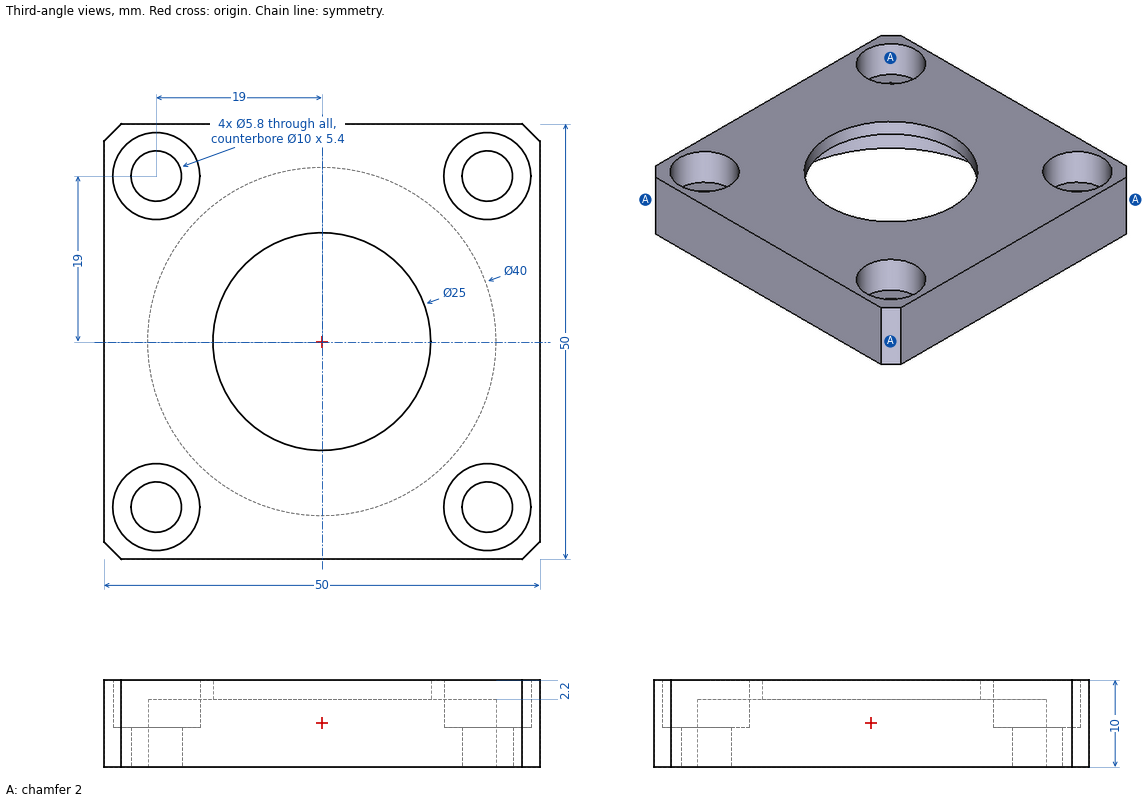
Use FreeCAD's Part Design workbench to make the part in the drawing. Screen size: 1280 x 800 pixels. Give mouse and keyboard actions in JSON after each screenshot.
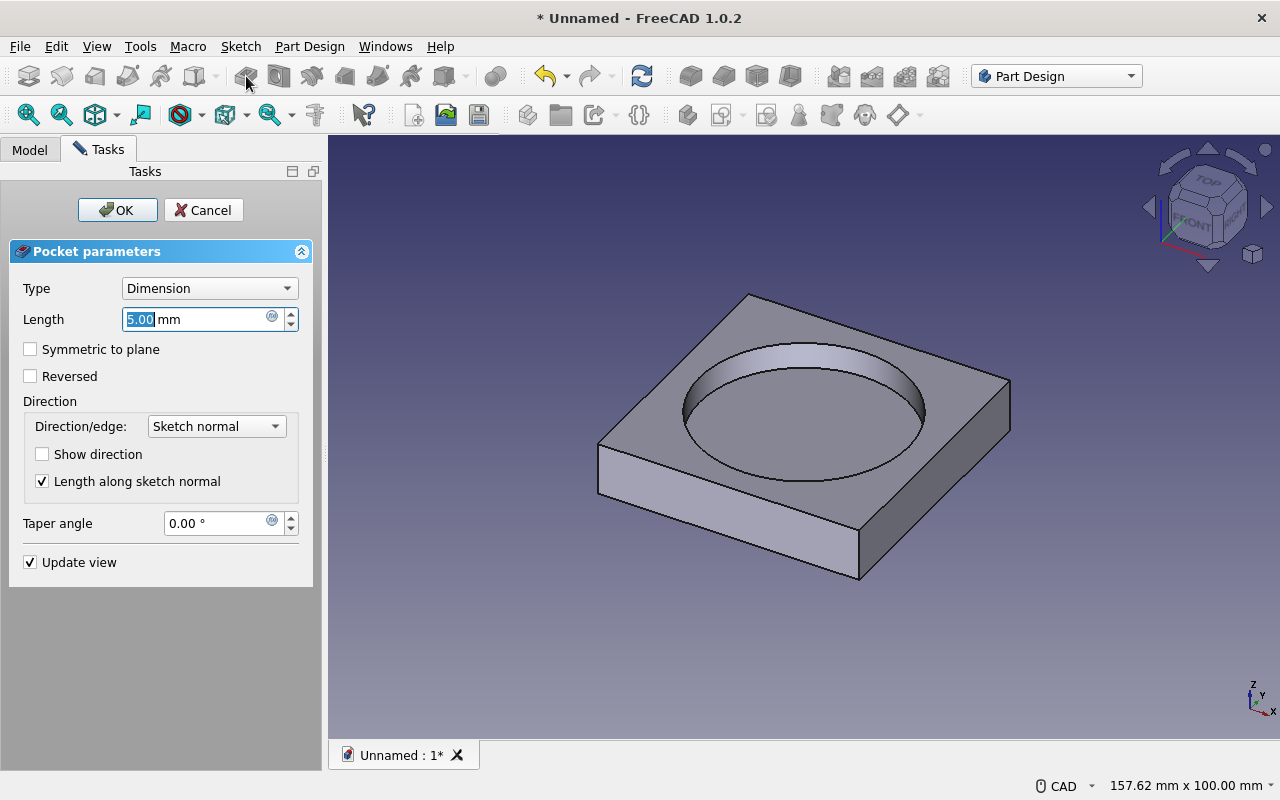
{"action": "left_click", "coordinate": [210, 288]}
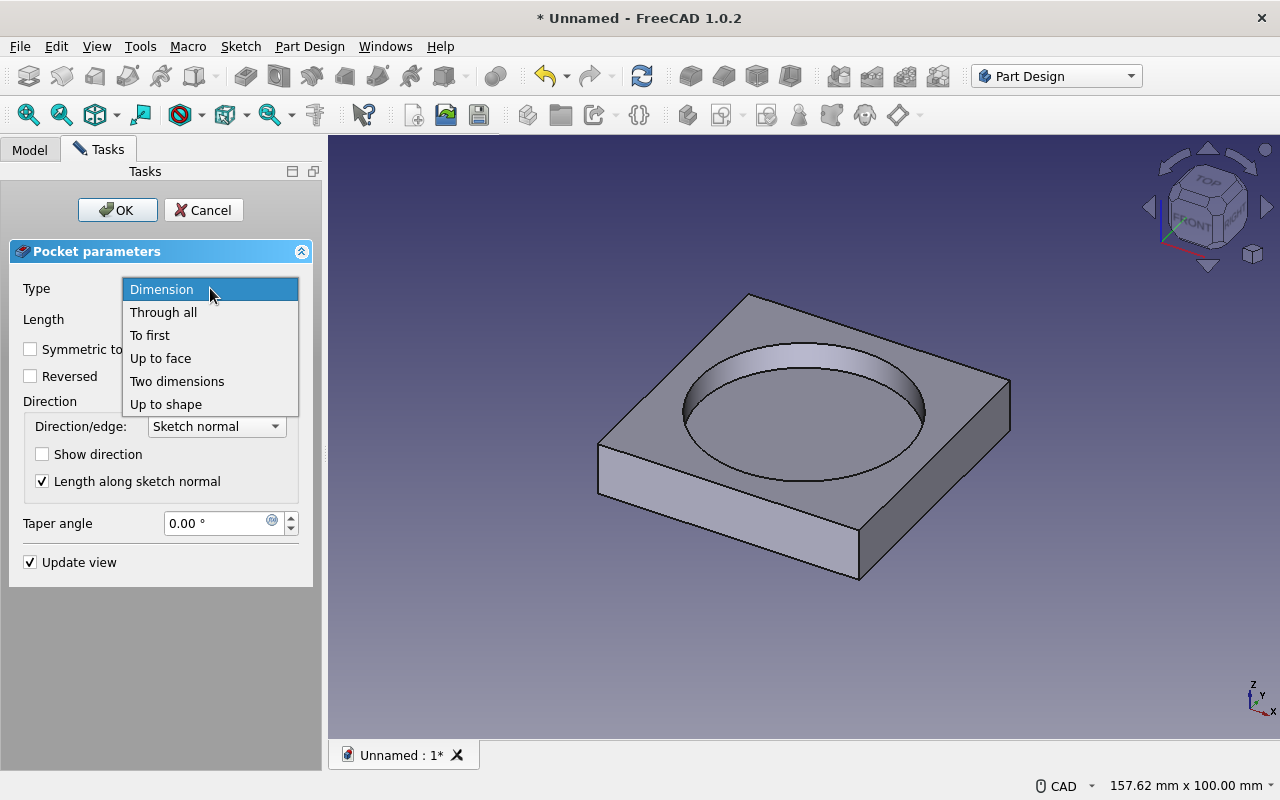
{"action": "left_click", "coordinate": [208, 312]}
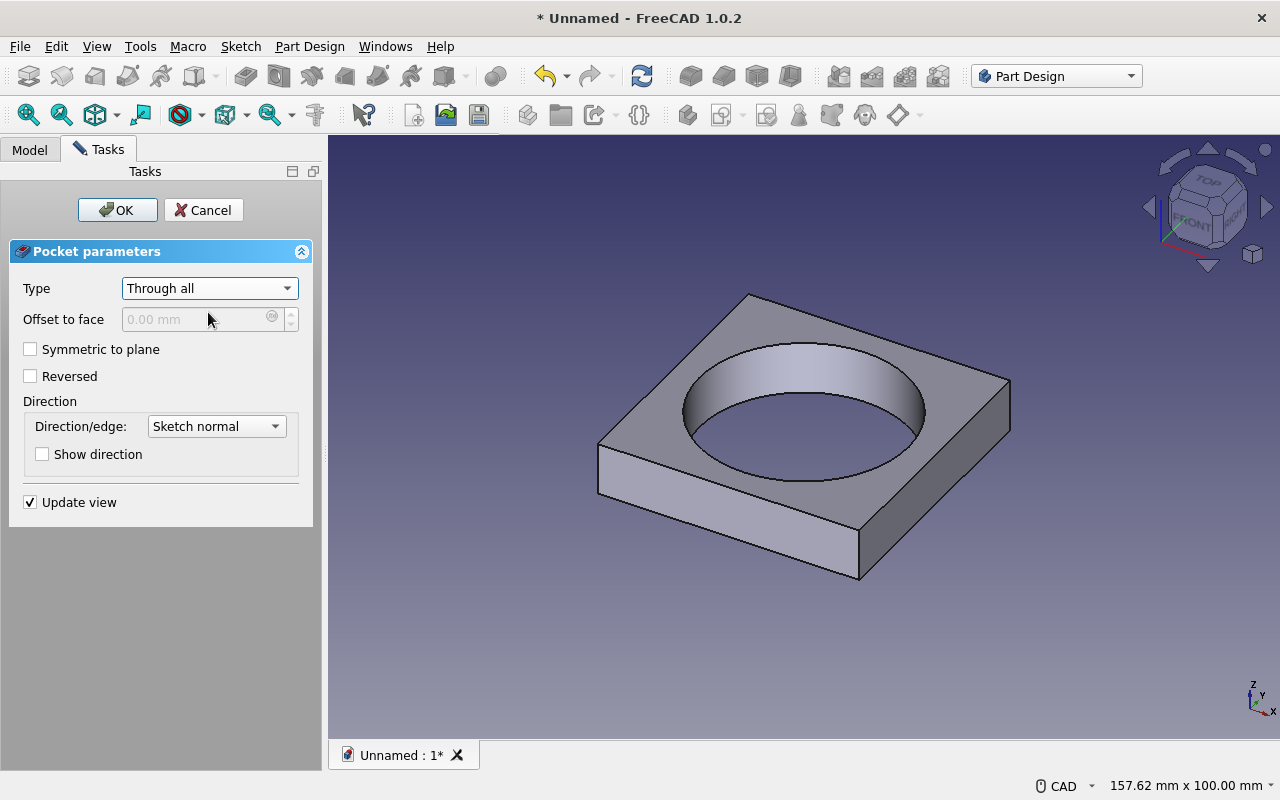
{"action": "left_click", "coordinate": [118, 210]}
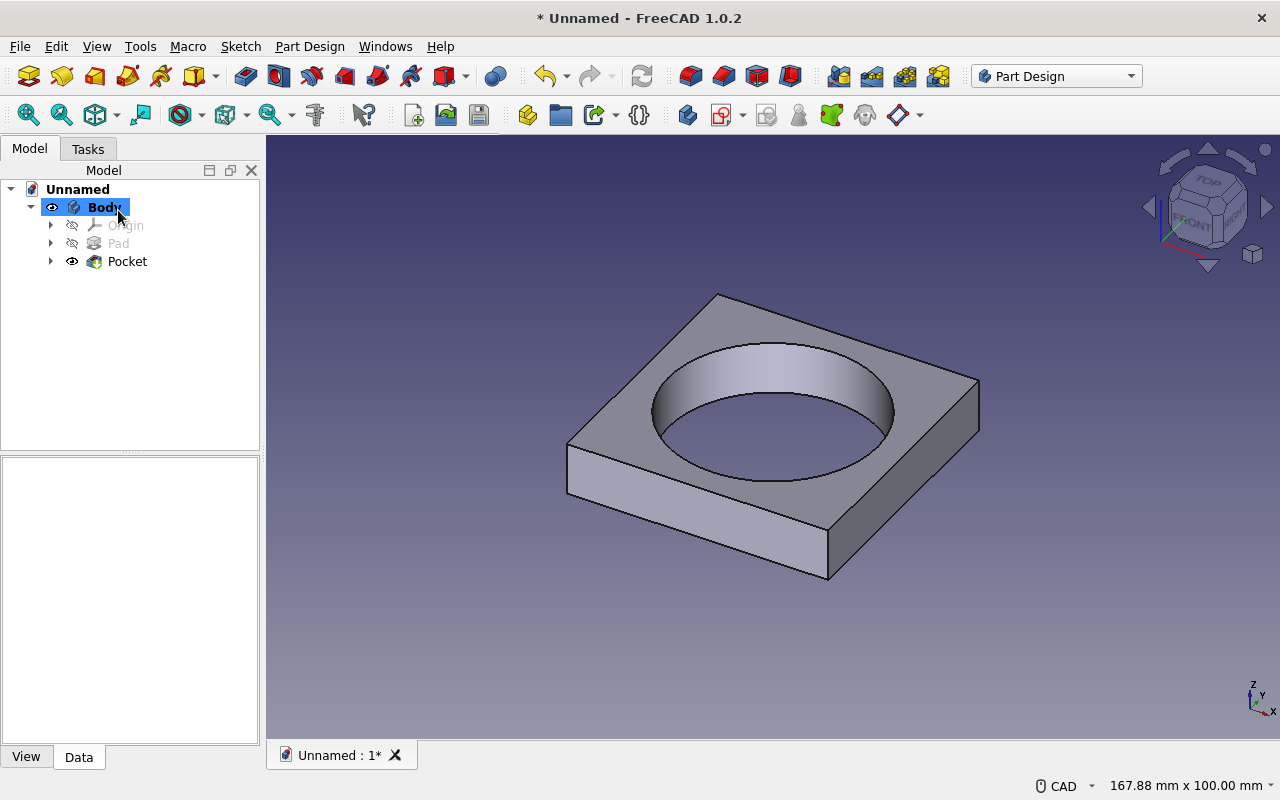
{"action": "left_click", "coordinate": [783, 500]}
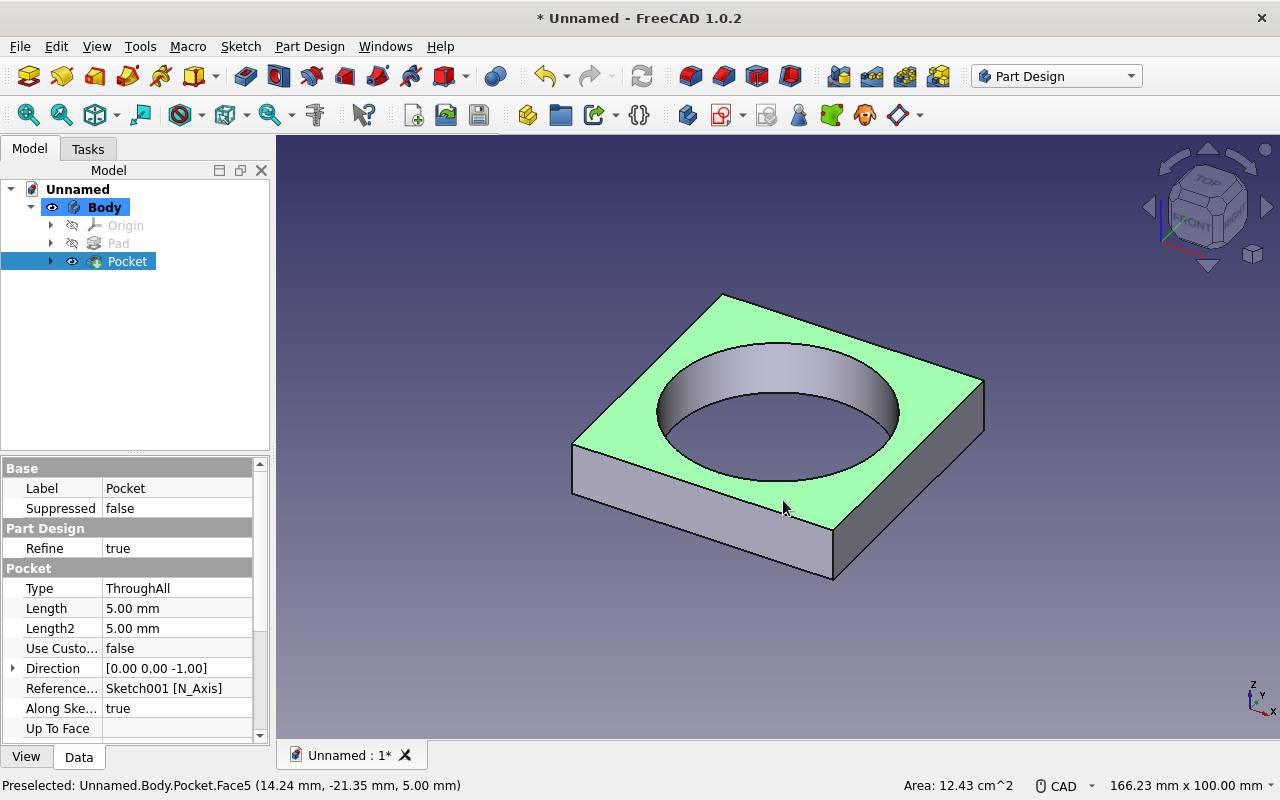
{"action": "left_click", "coordinate": [720, 116]}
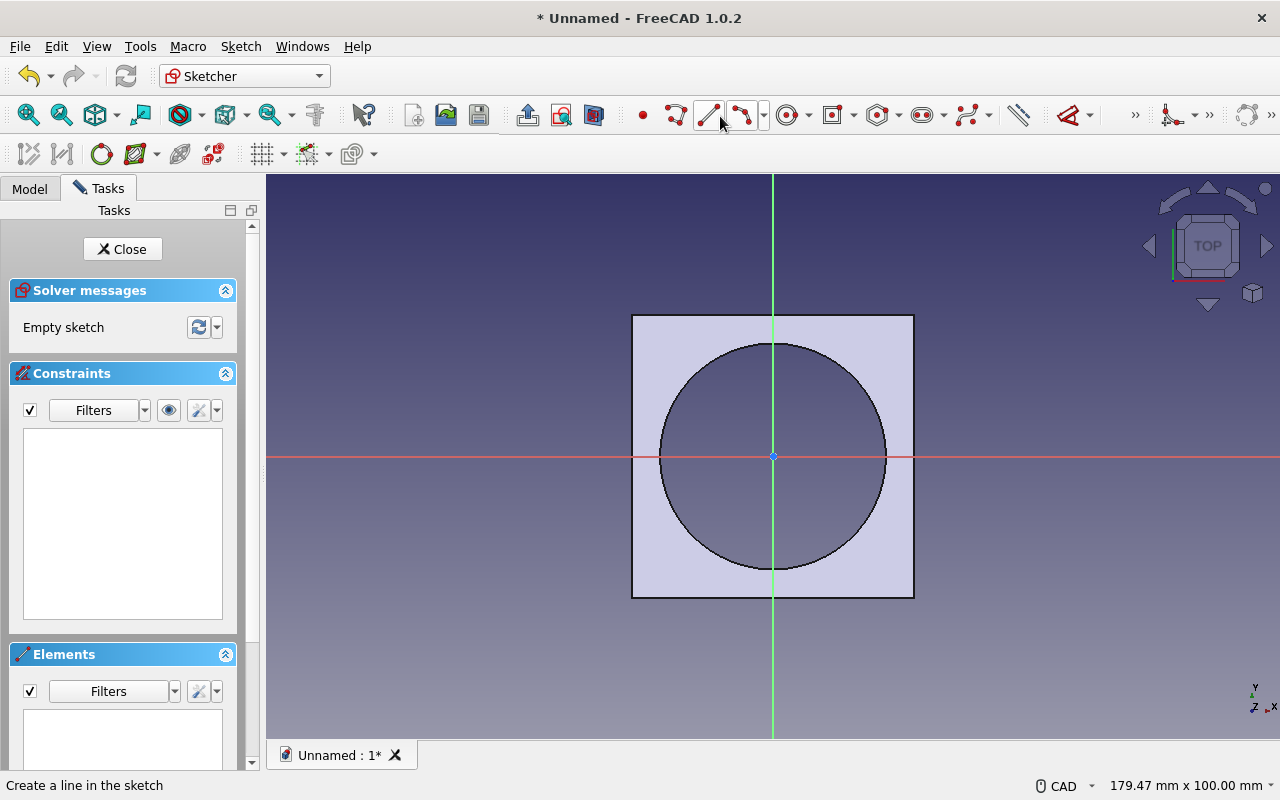
{"action": "scroll", "coordinate": [912, 456], "scroll_direction": "up", "scroll_amount": 2}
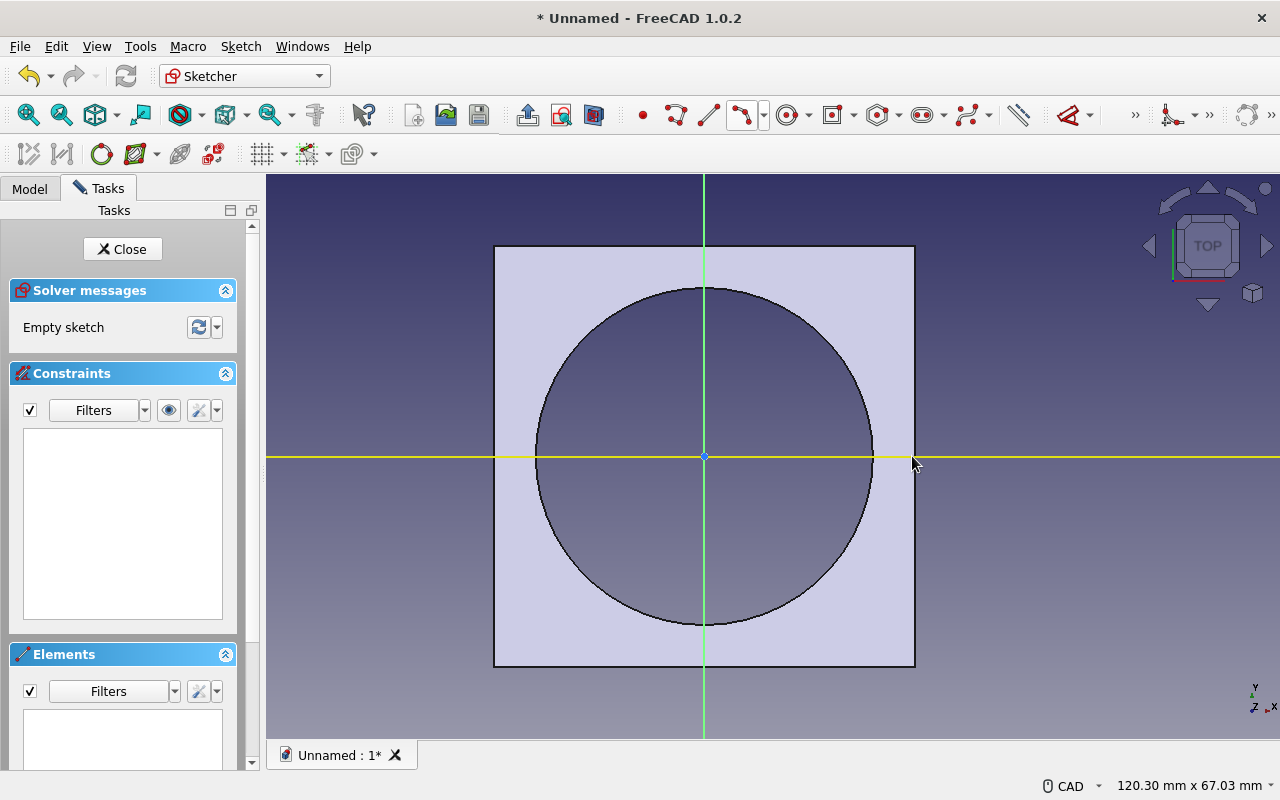
{"action": "left_click", "coordinate": [786, 116]}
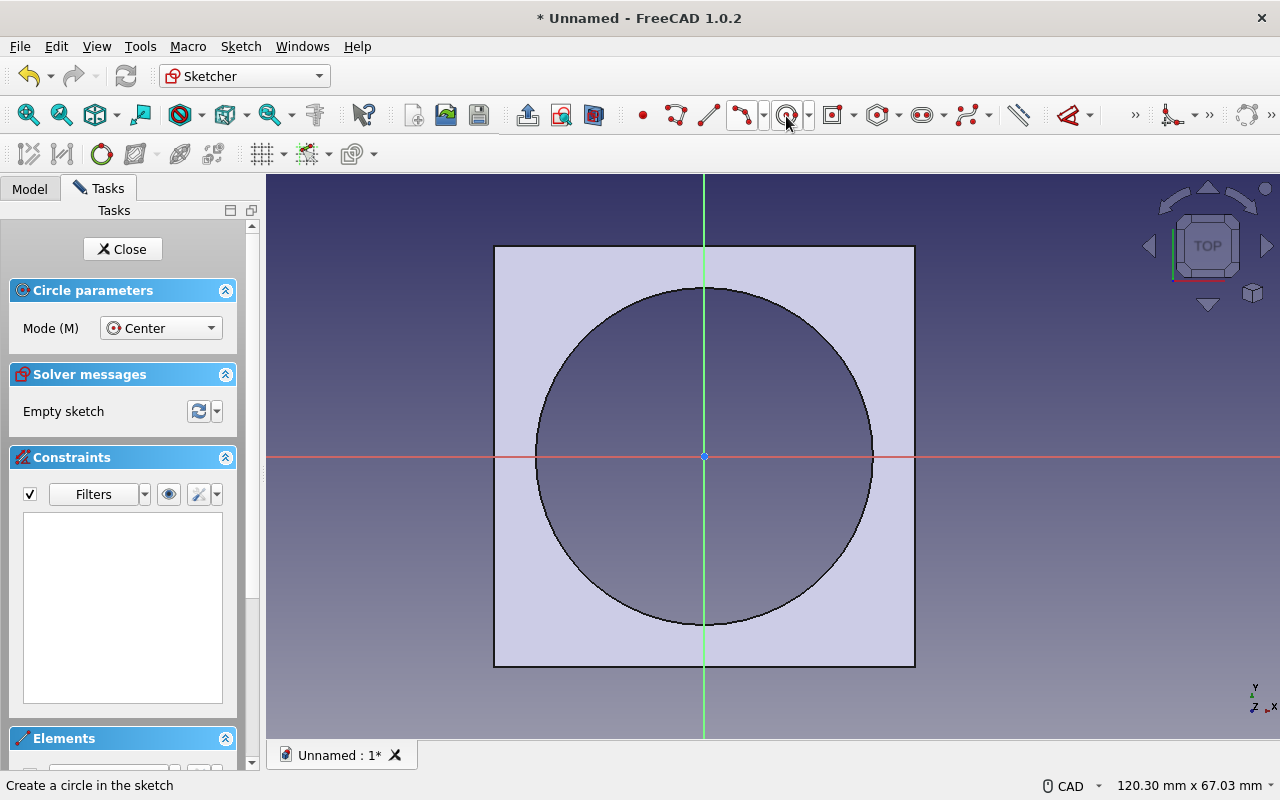
{"action": "left_click", "coordinate": [544, 296]}
{"action": "mouse_move", "coordinate": [561, 279]}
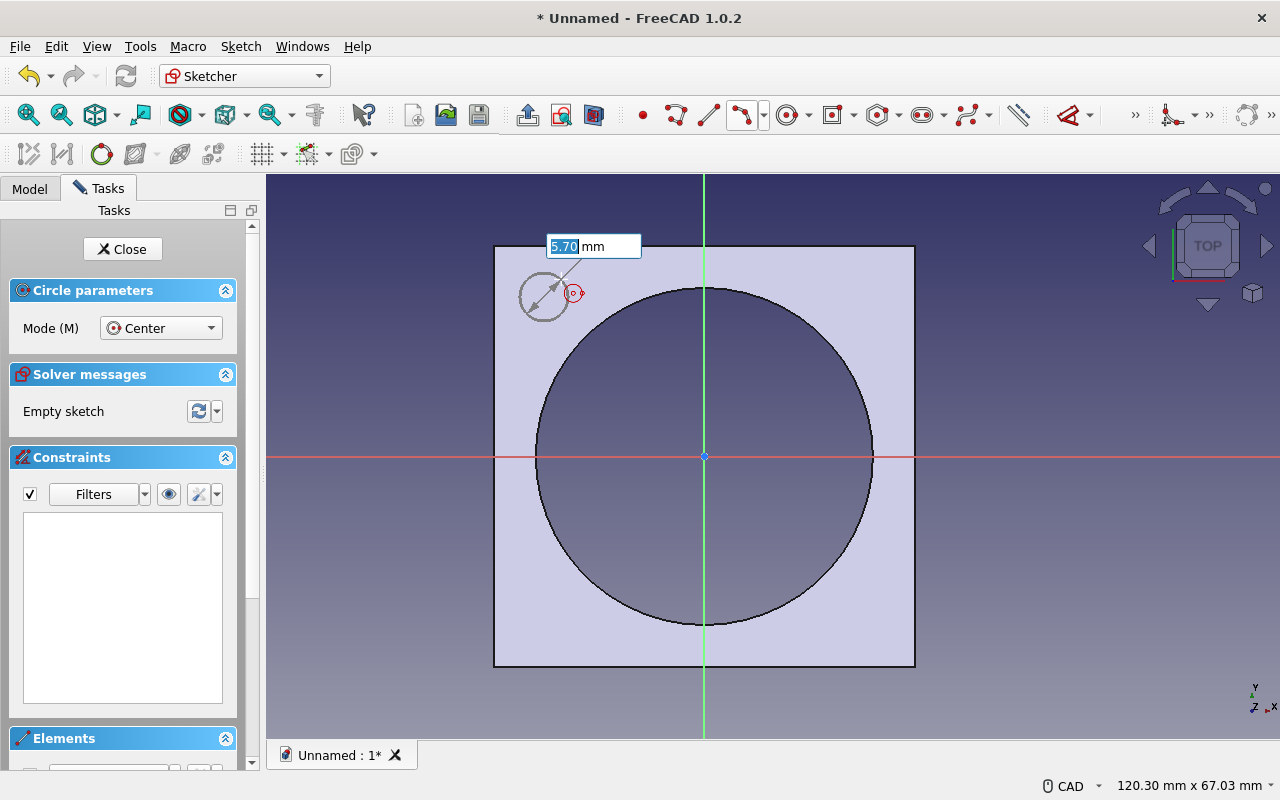
{"action": "type", "text": "5.8"}
{"action": "key", "text": "Return"}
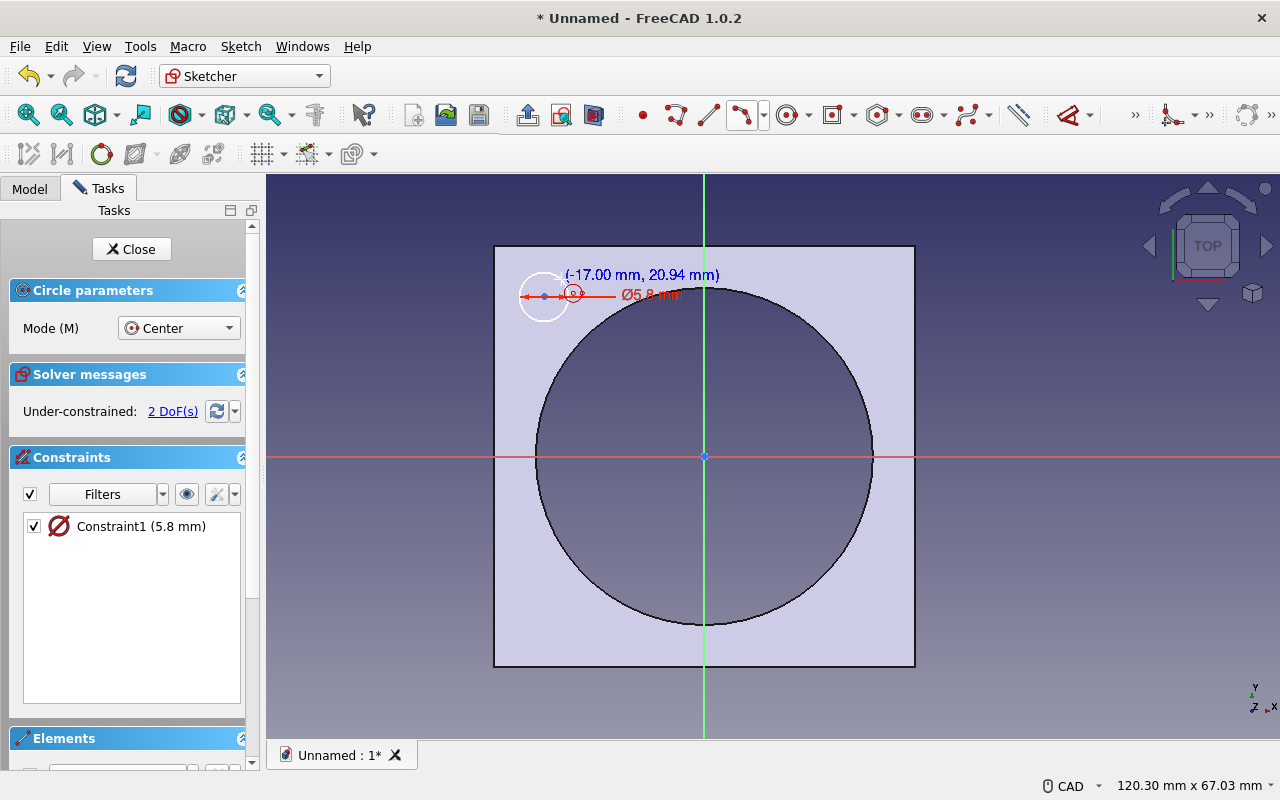
{"action": "left_click", "coordinate": [864, 296]}
{"action": "mouse_move", "coordinate": [882, 279]}